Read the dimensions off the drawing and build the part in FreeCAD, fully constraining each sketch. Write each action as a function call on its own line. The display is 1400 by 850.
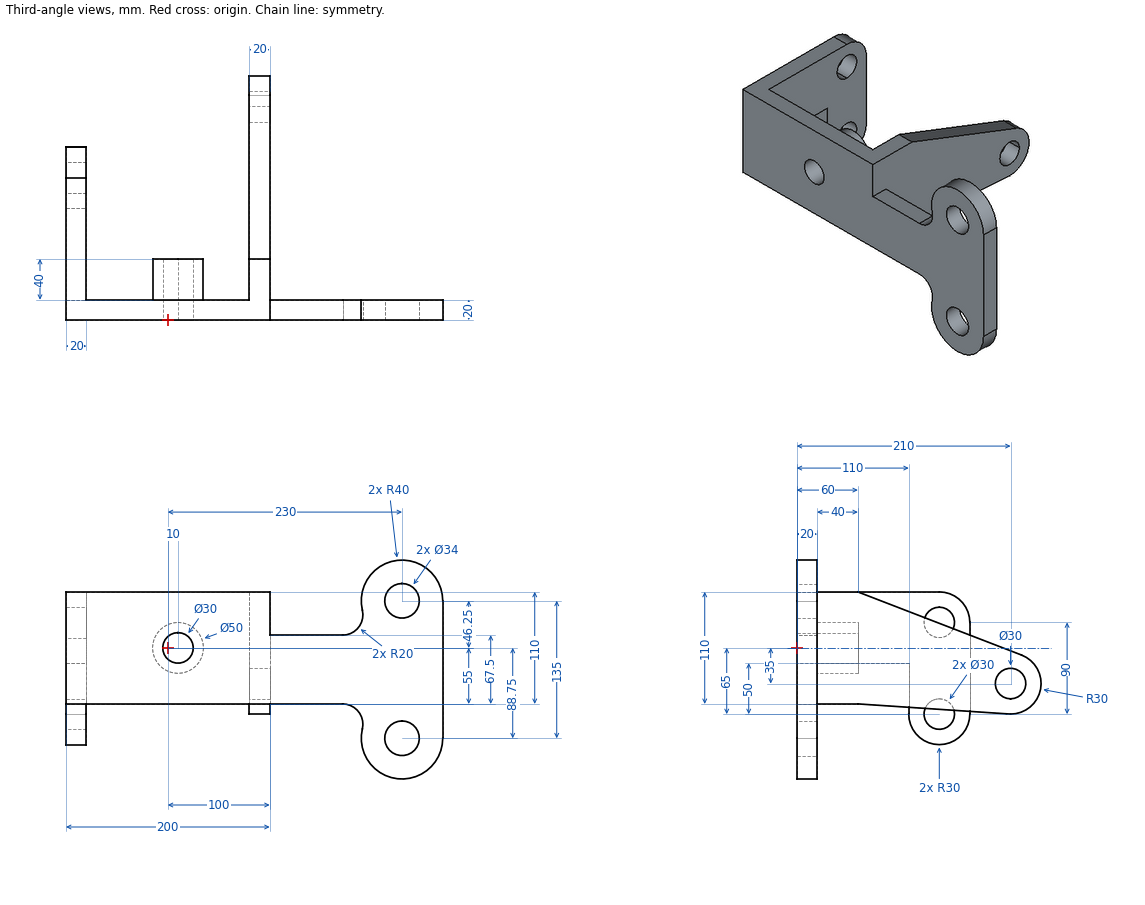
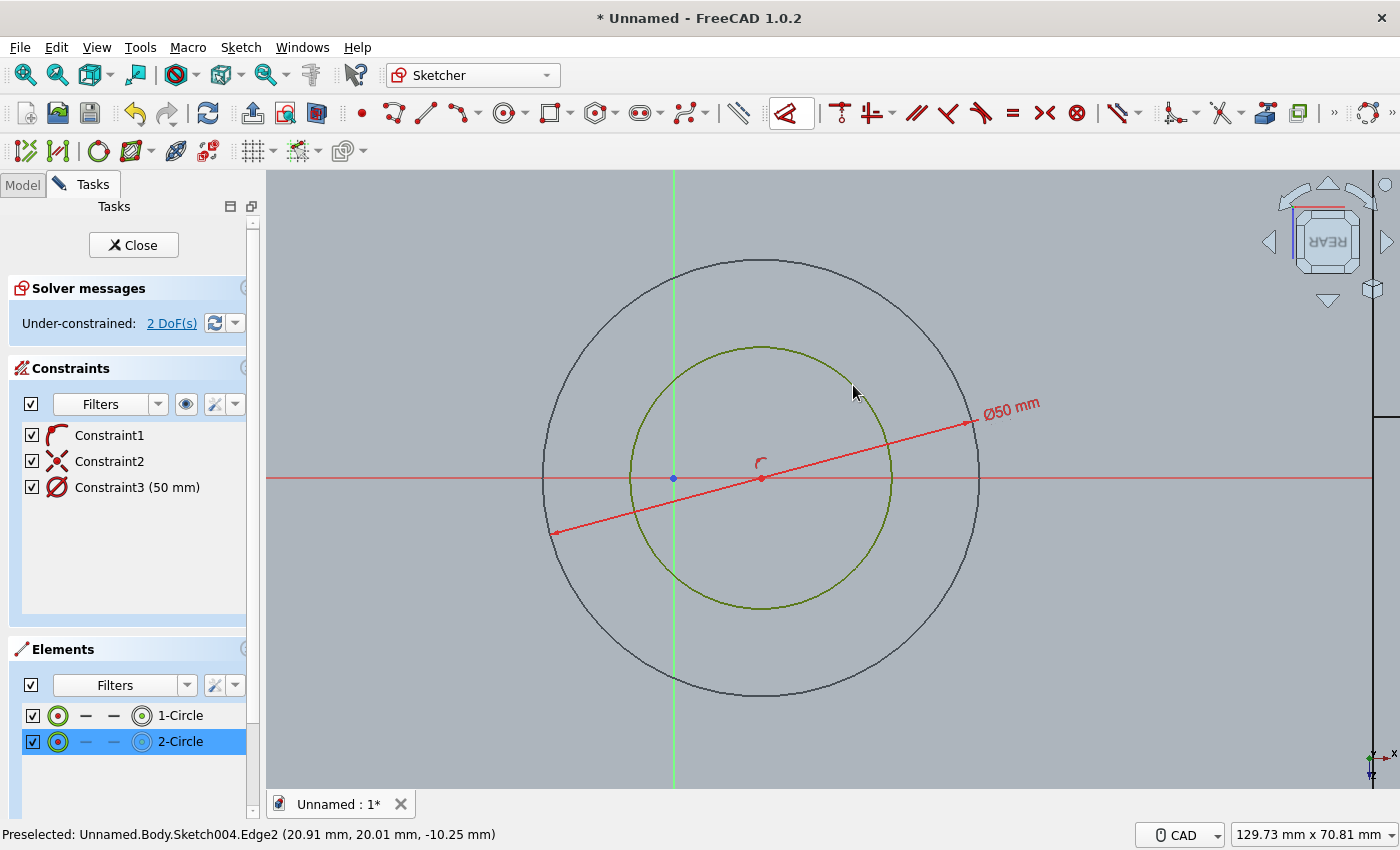
click(808, 114)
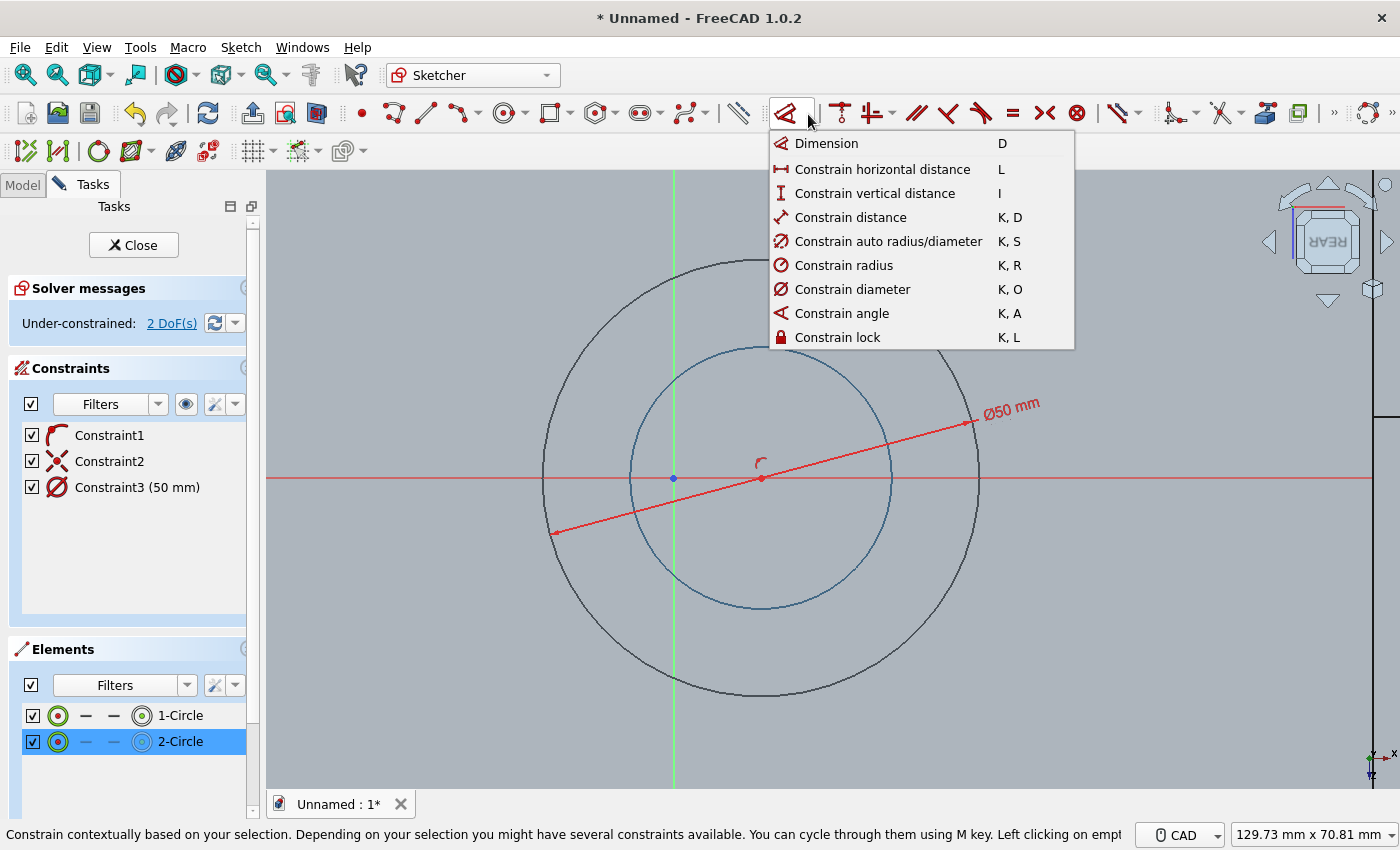
click(922, 289)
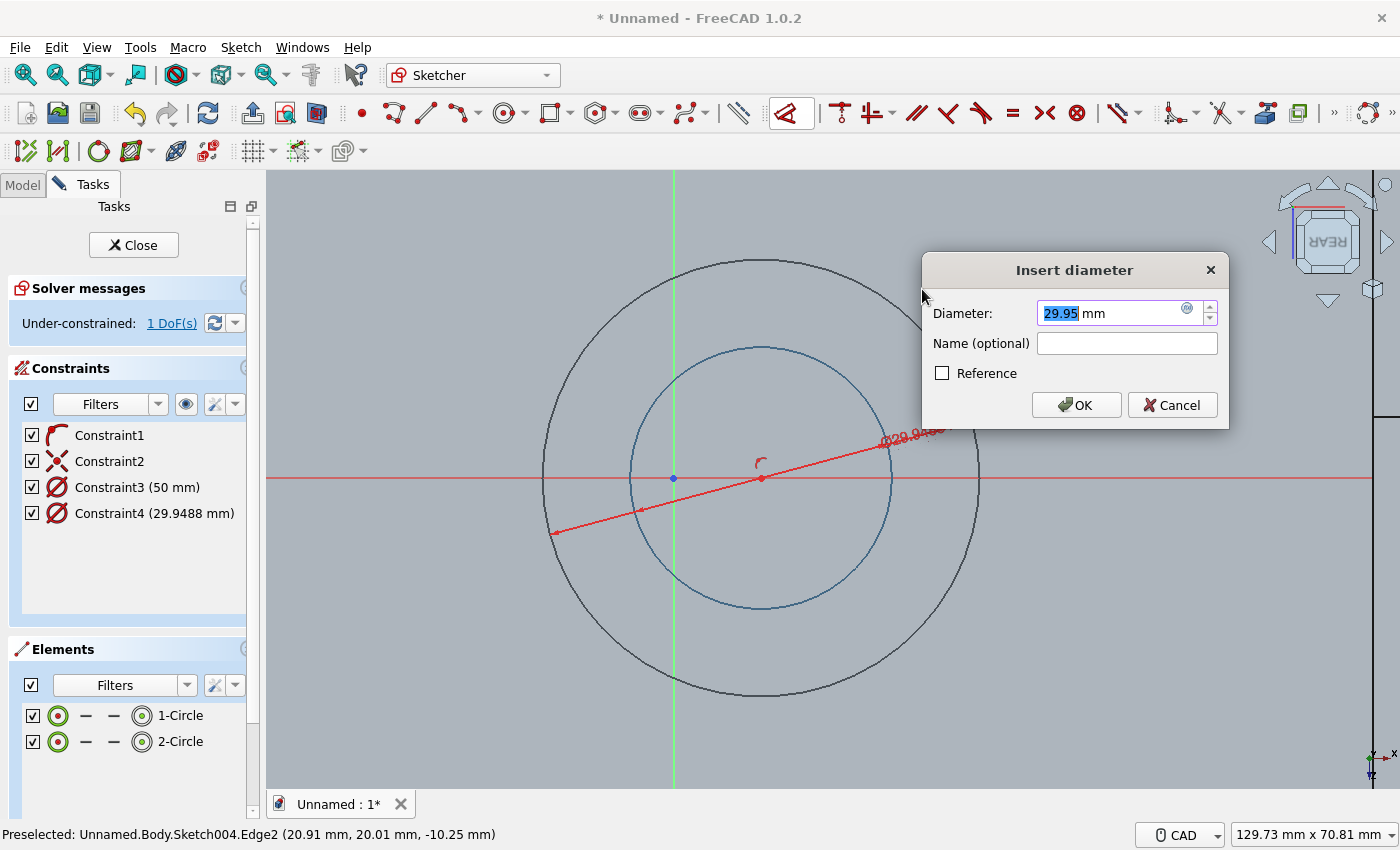
text(30)
key(Return)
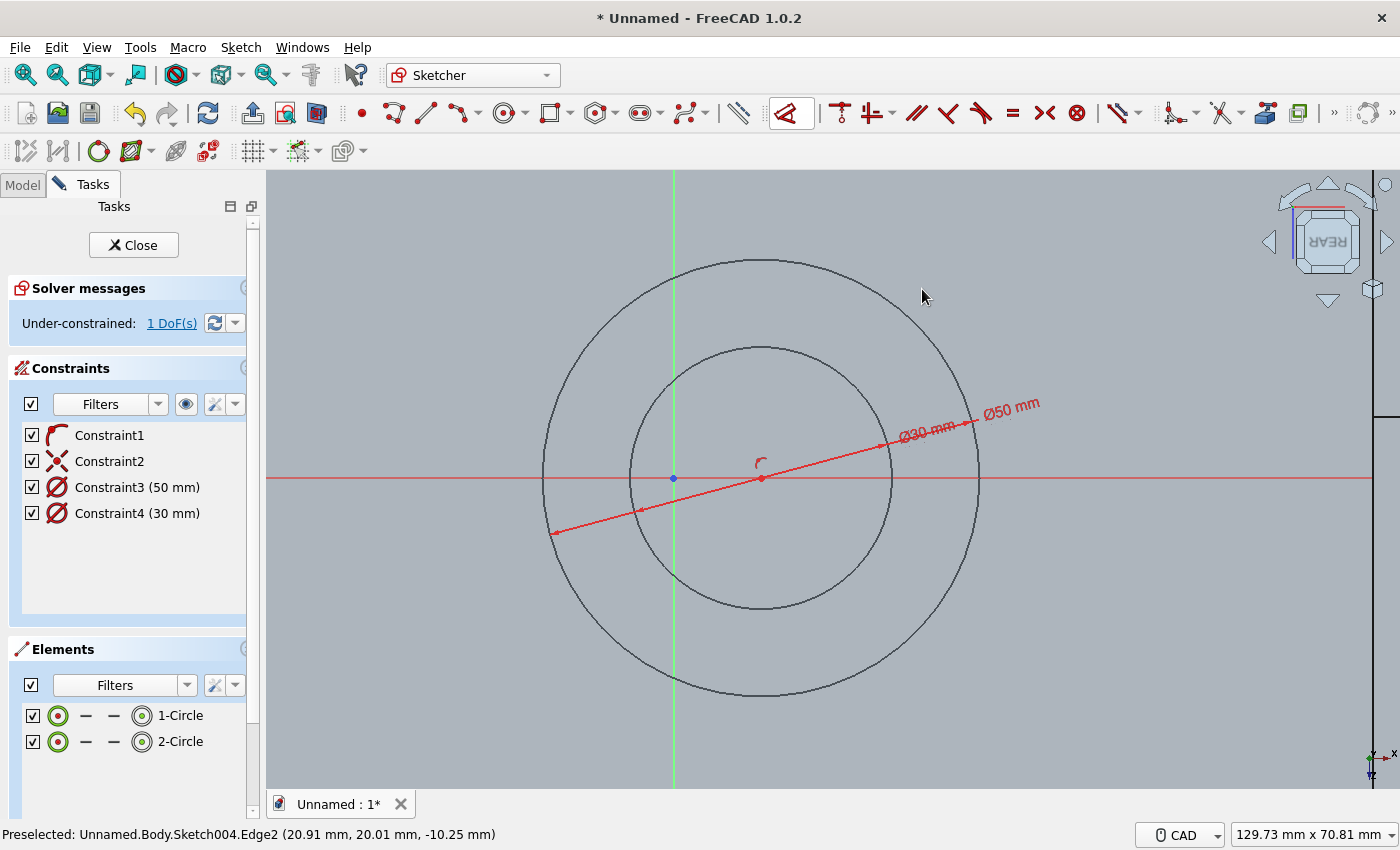
click(761, 478)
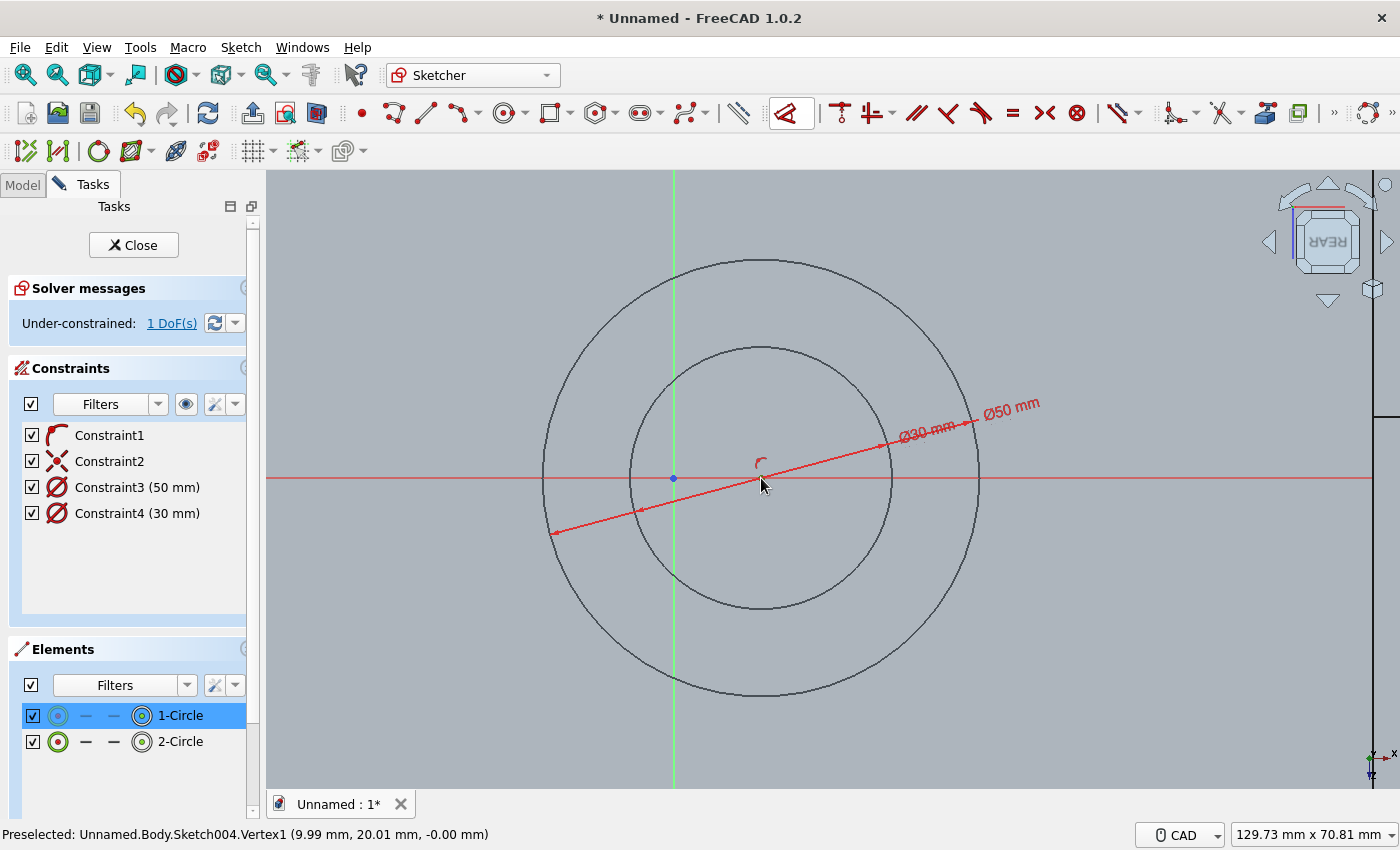
key(l)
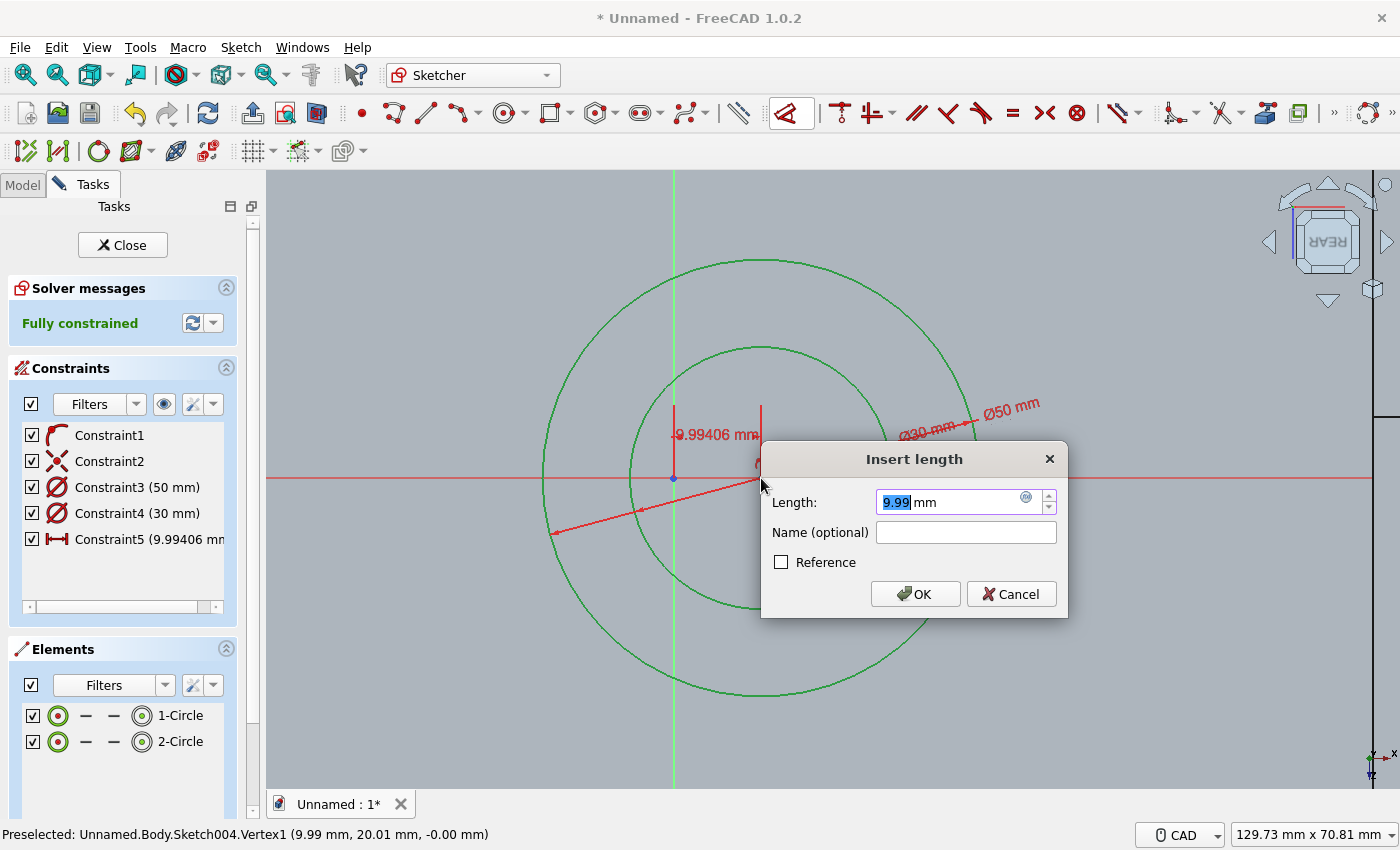
text(10)
key(Return)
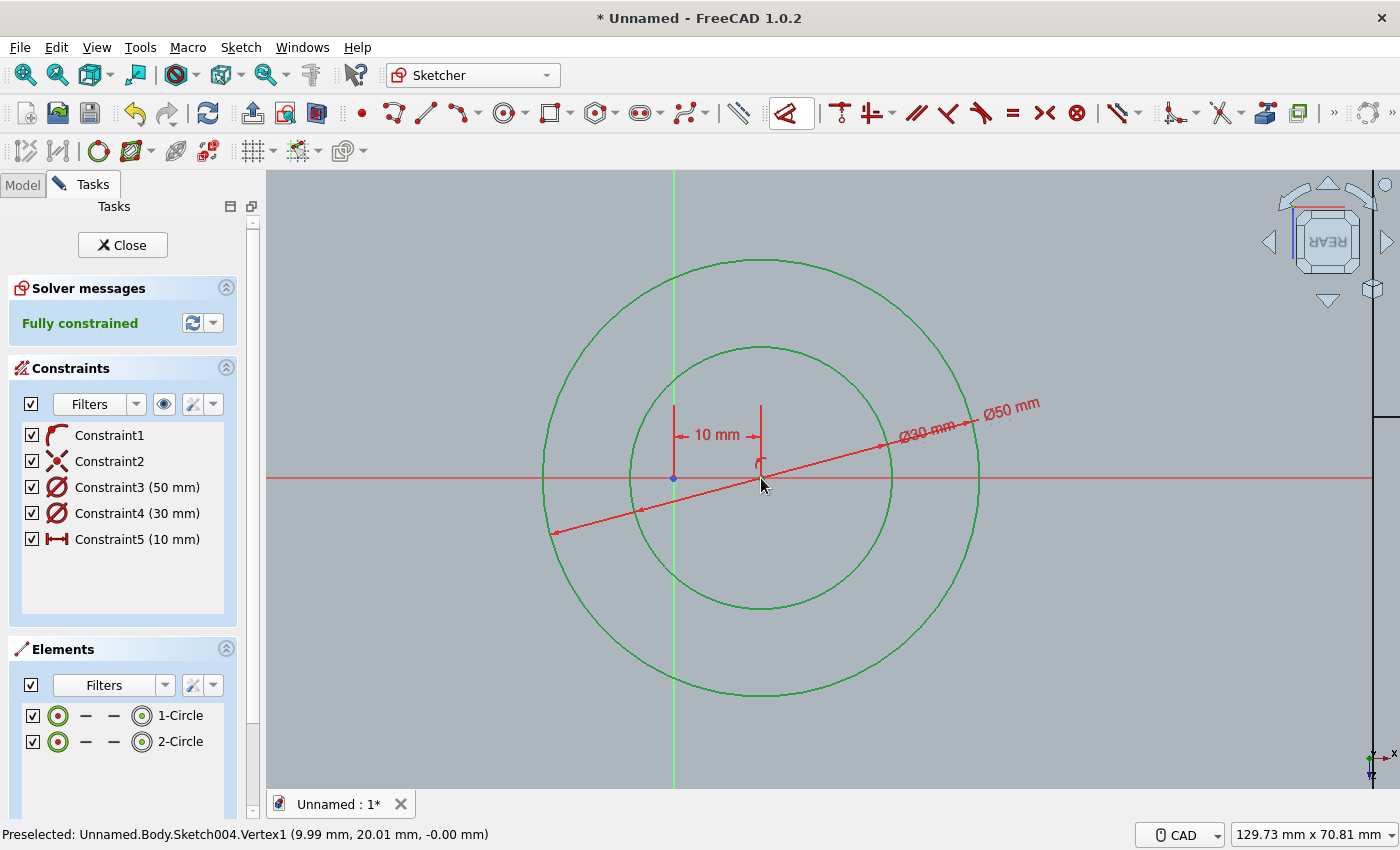
click(123, 245)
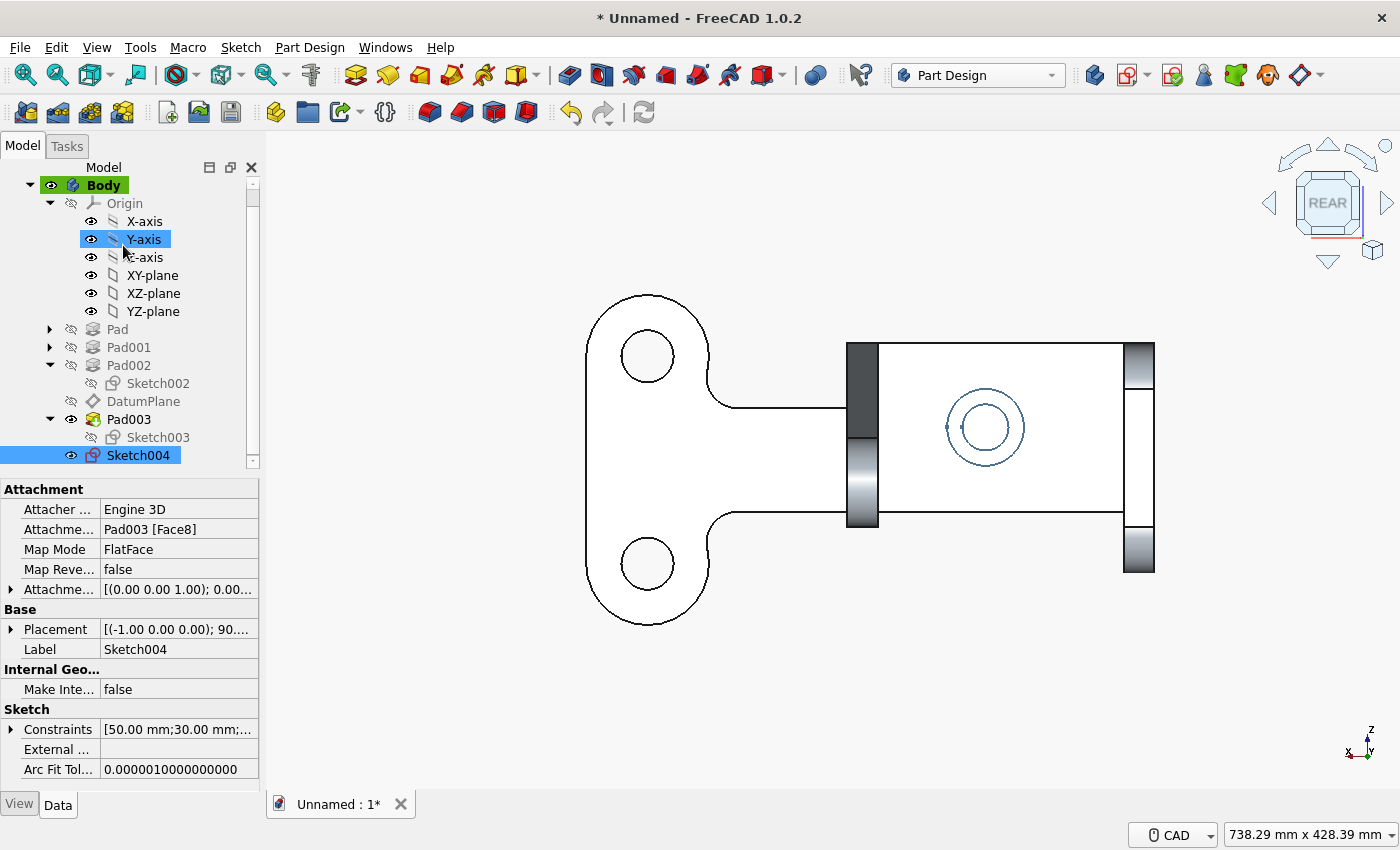
click(356, 76)